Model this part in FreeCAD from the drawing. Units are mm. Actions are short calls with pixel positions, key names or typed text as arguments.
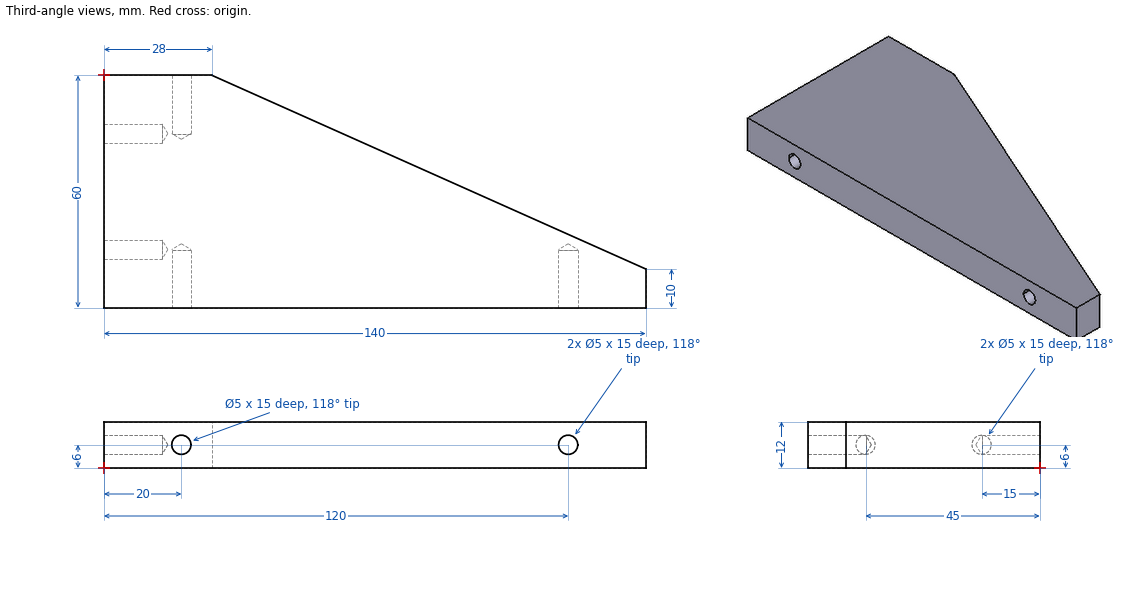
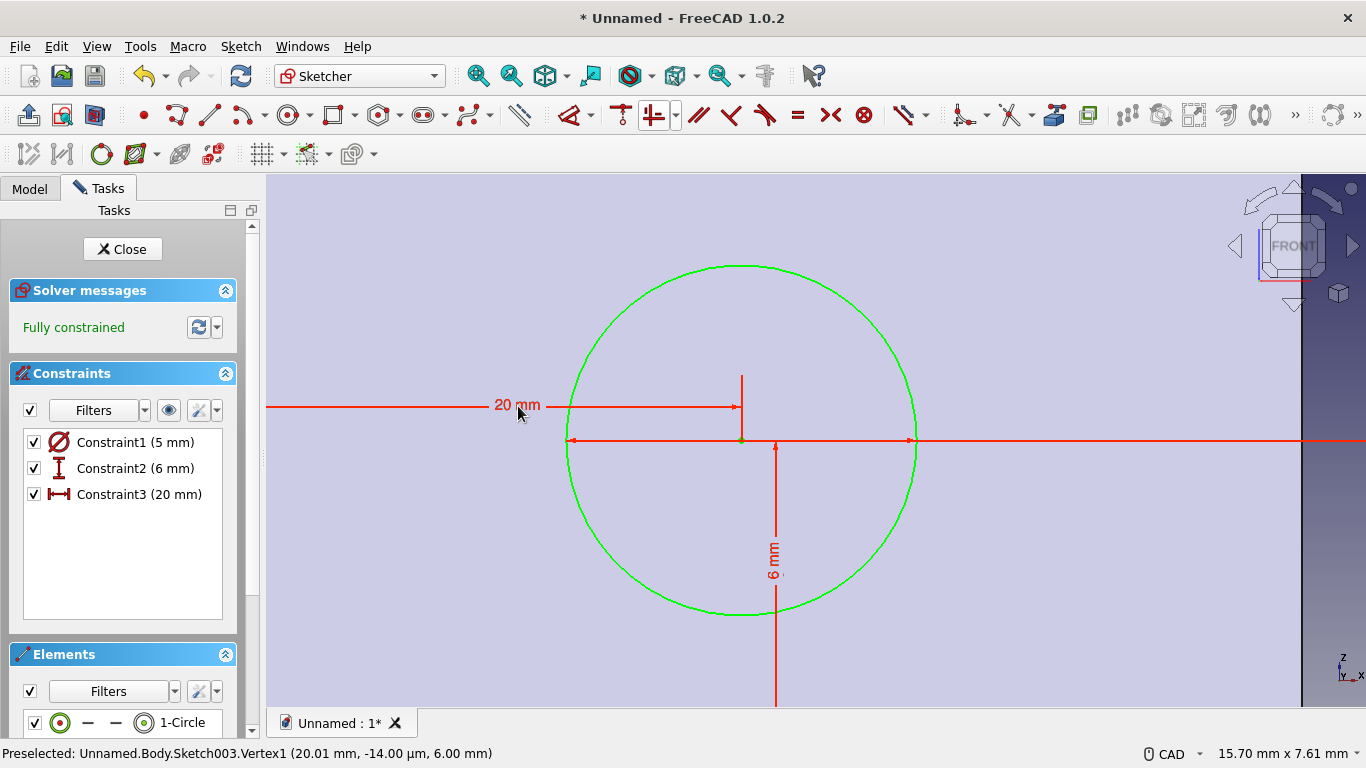
click(123, 249)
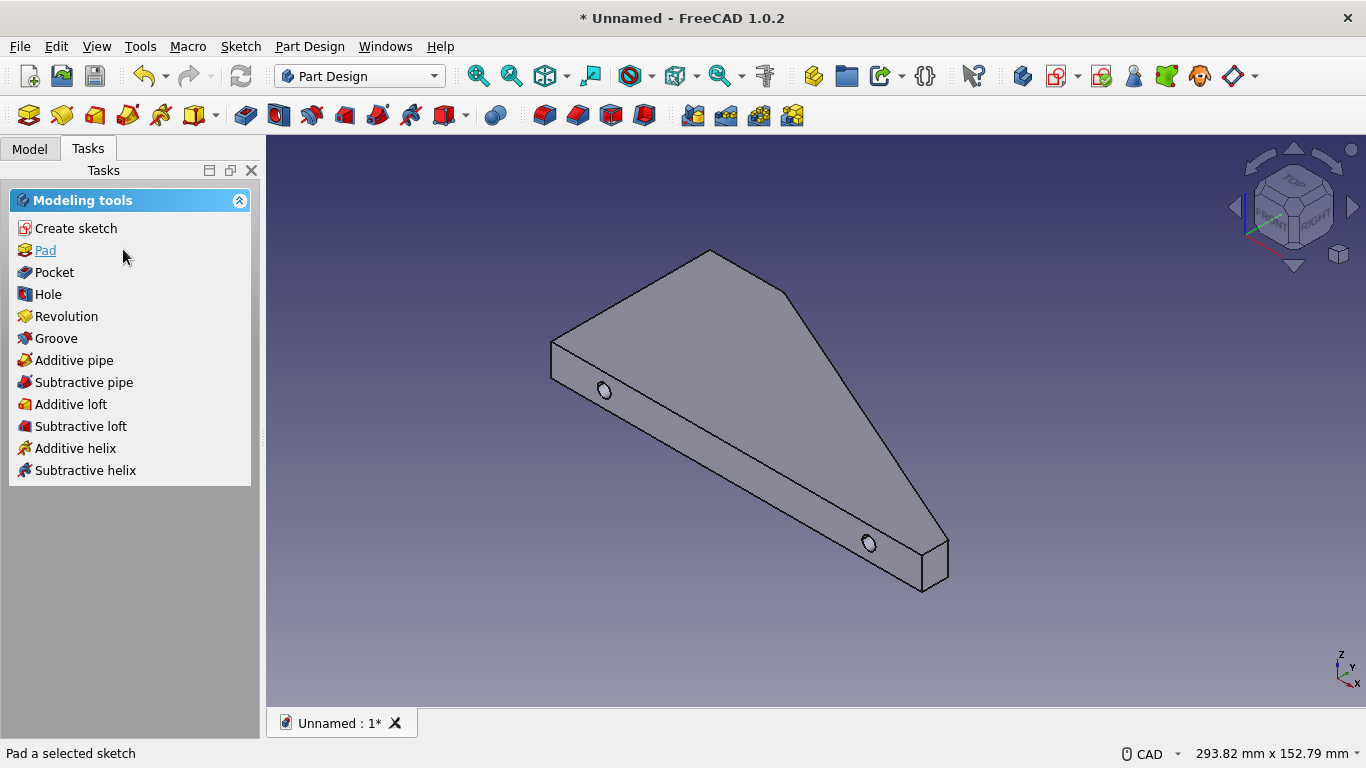
click(279, 116)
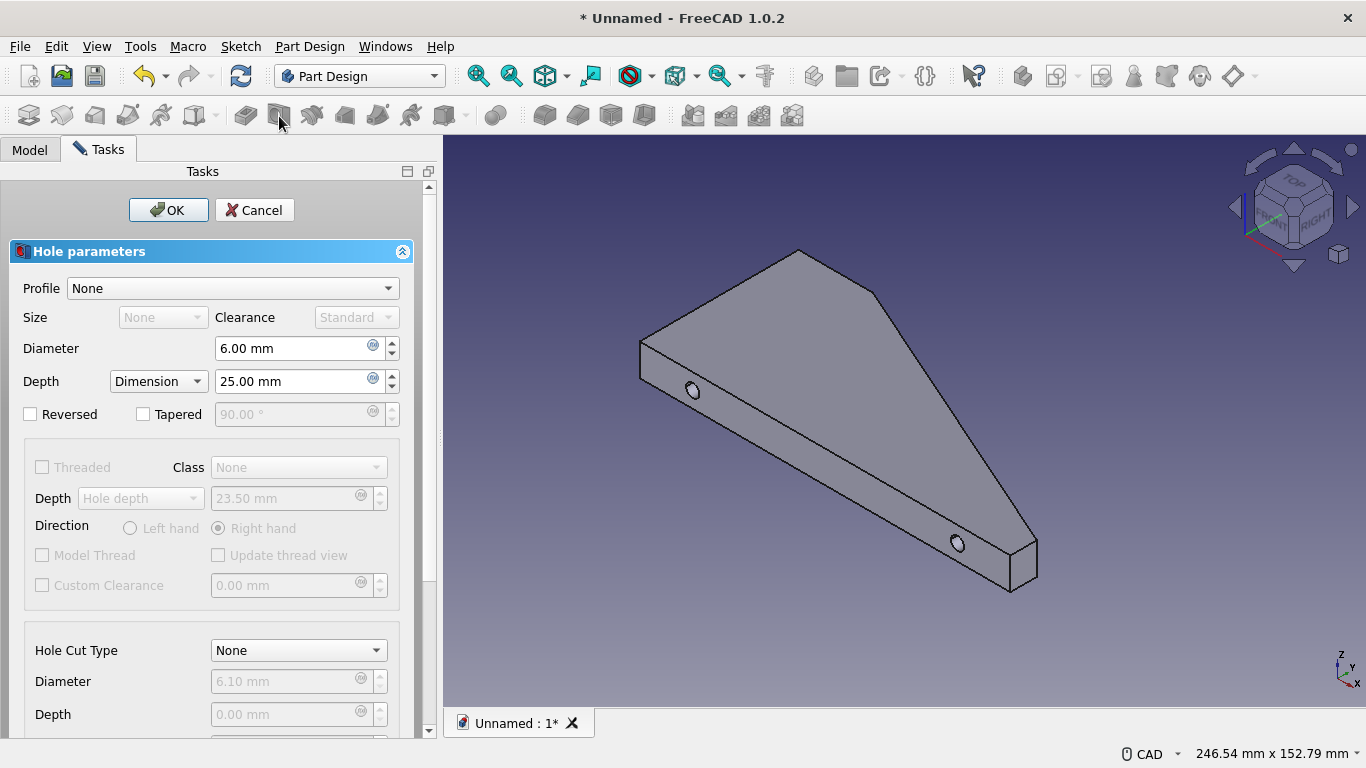
triple_click(300, 348)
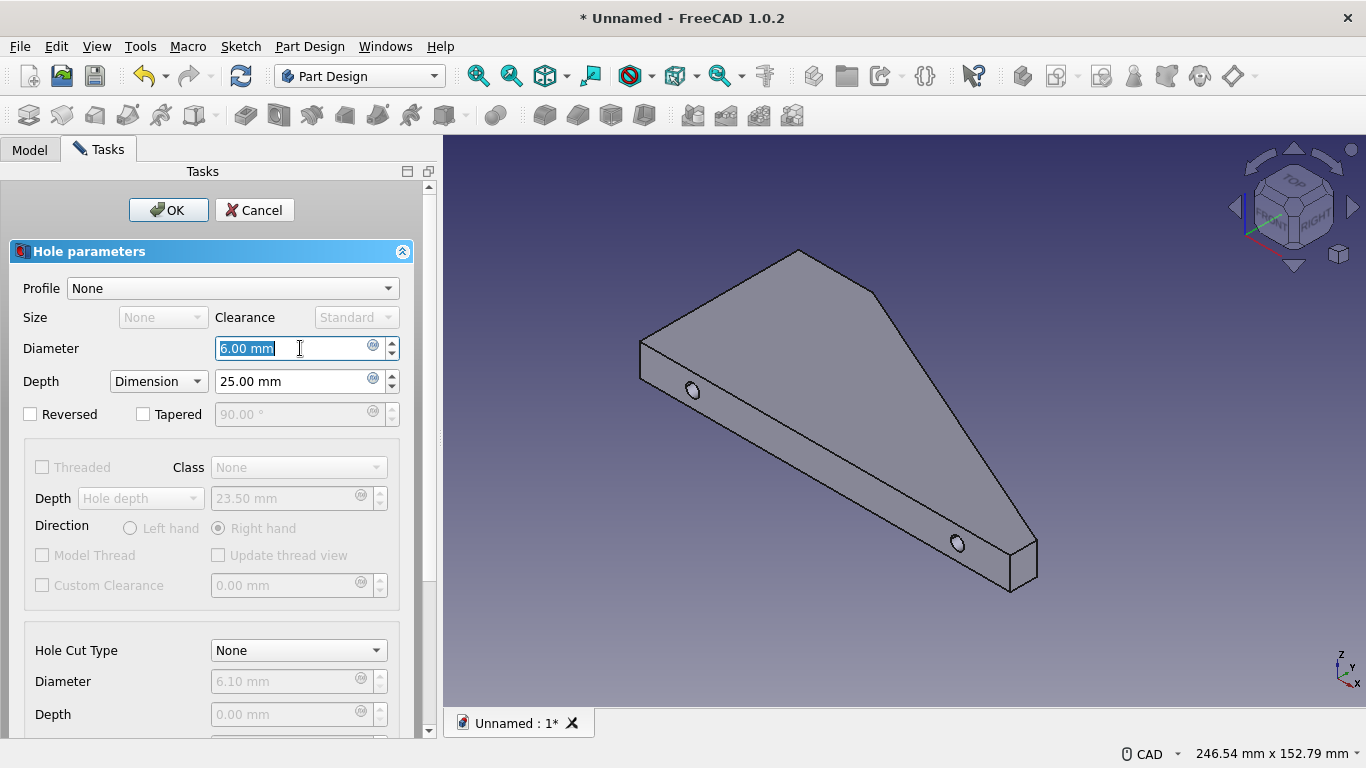
text(5)
key(Tab)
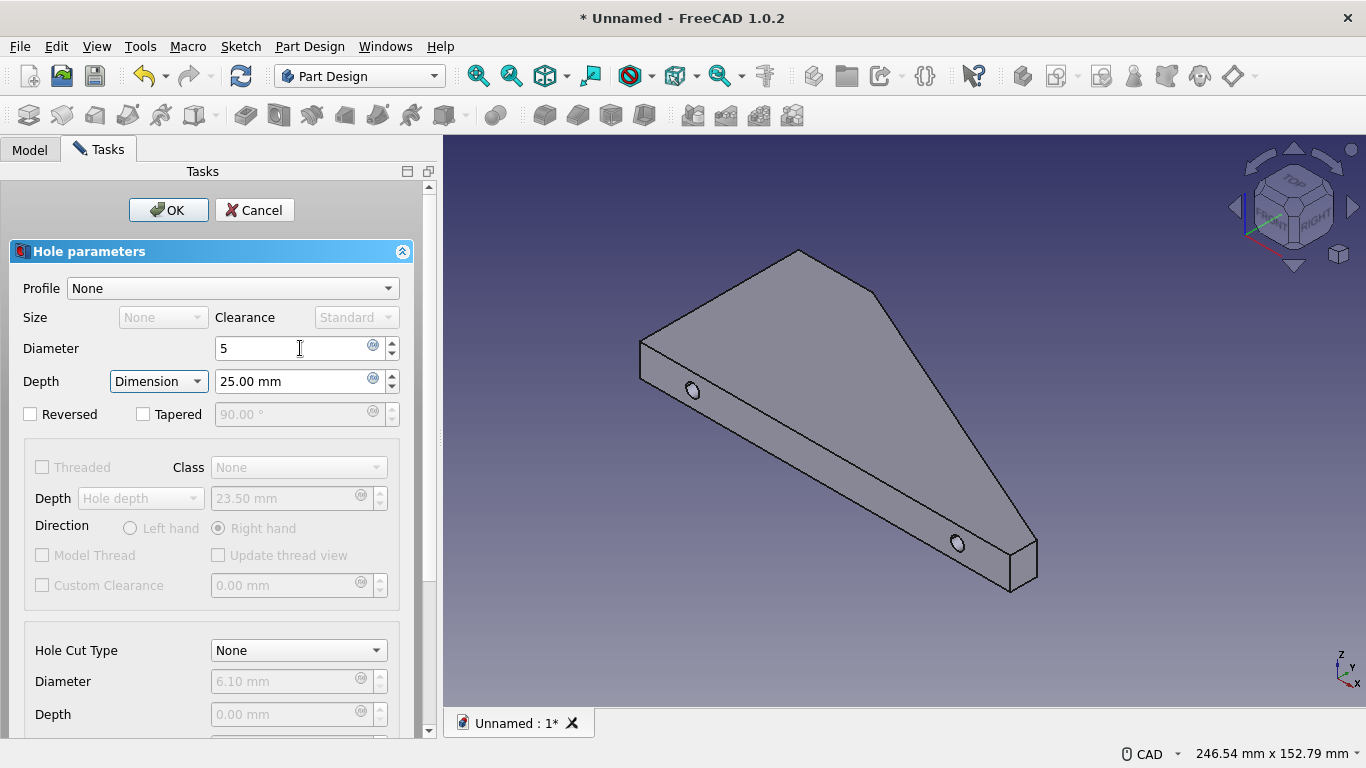
triple_click(300, 382)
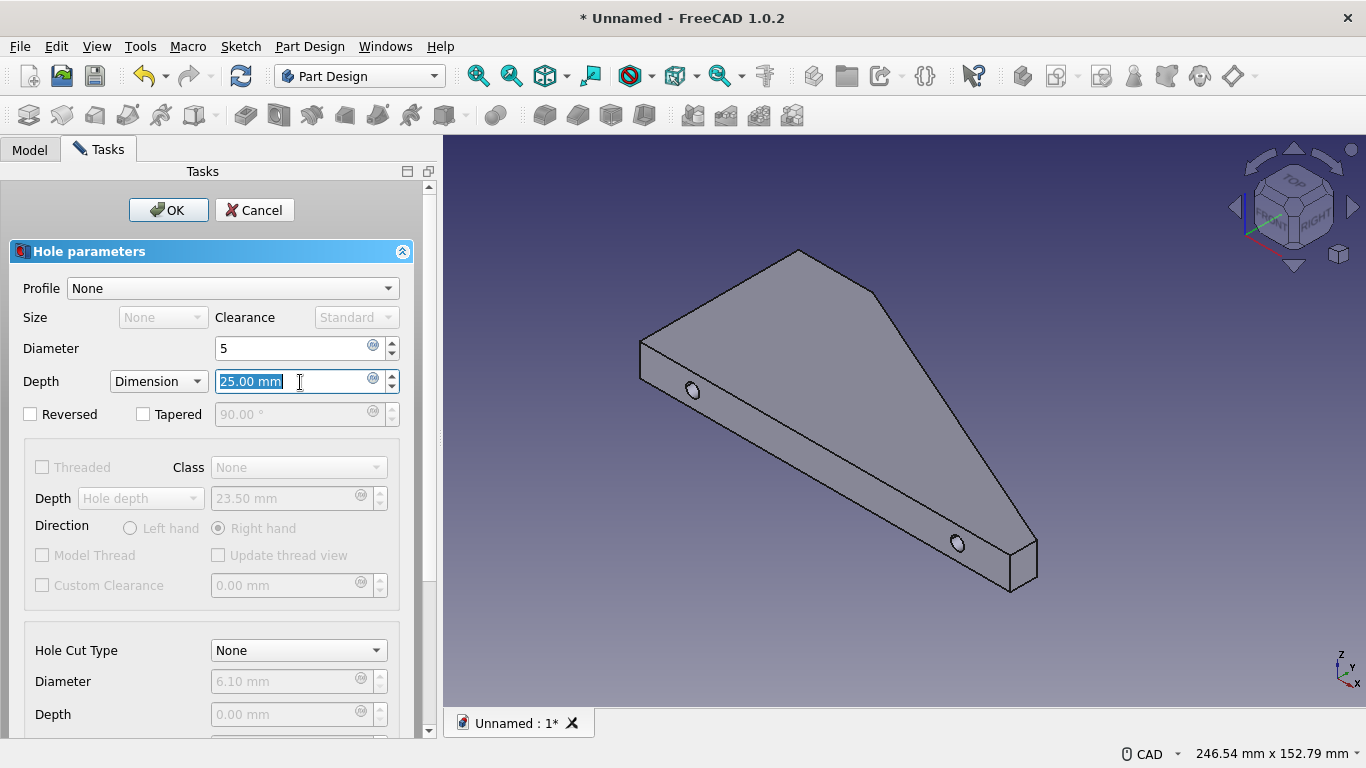
text(15)
key(Tab)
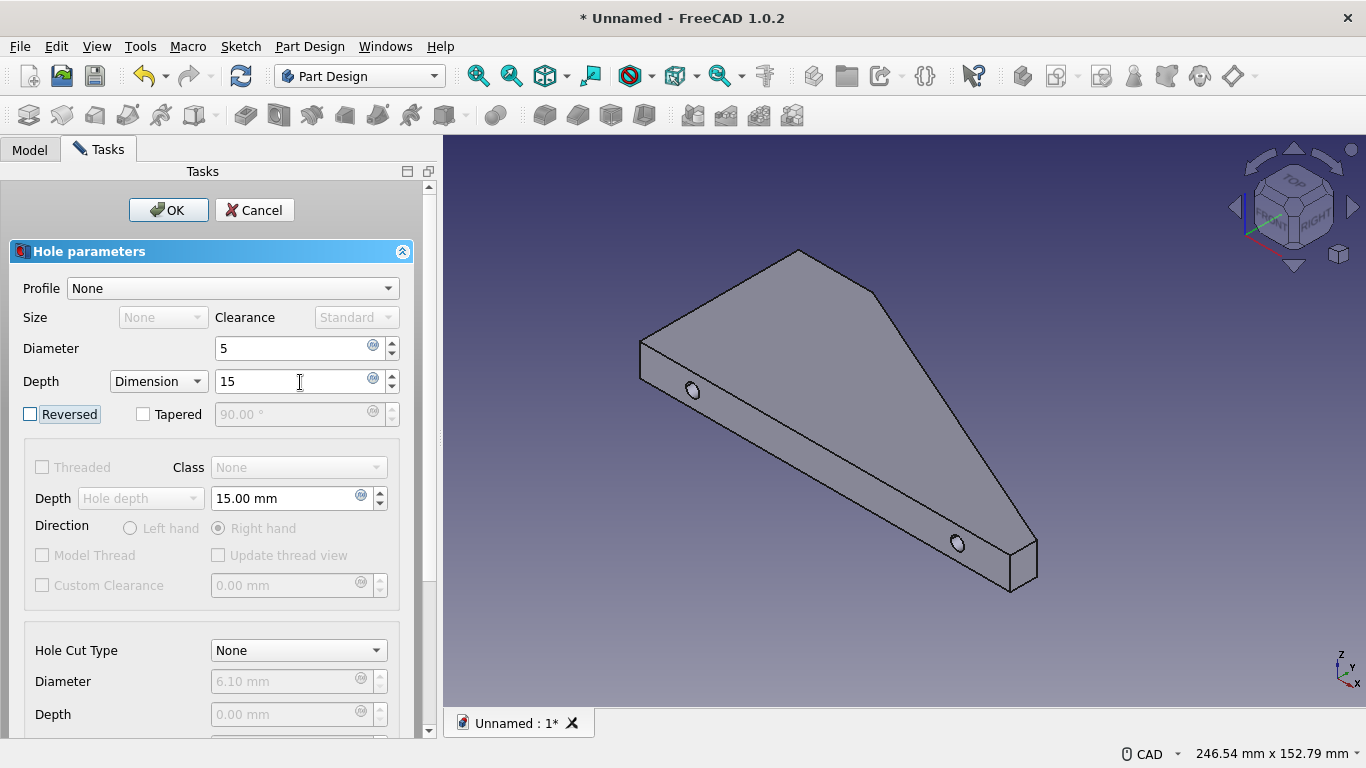
click(31, 414)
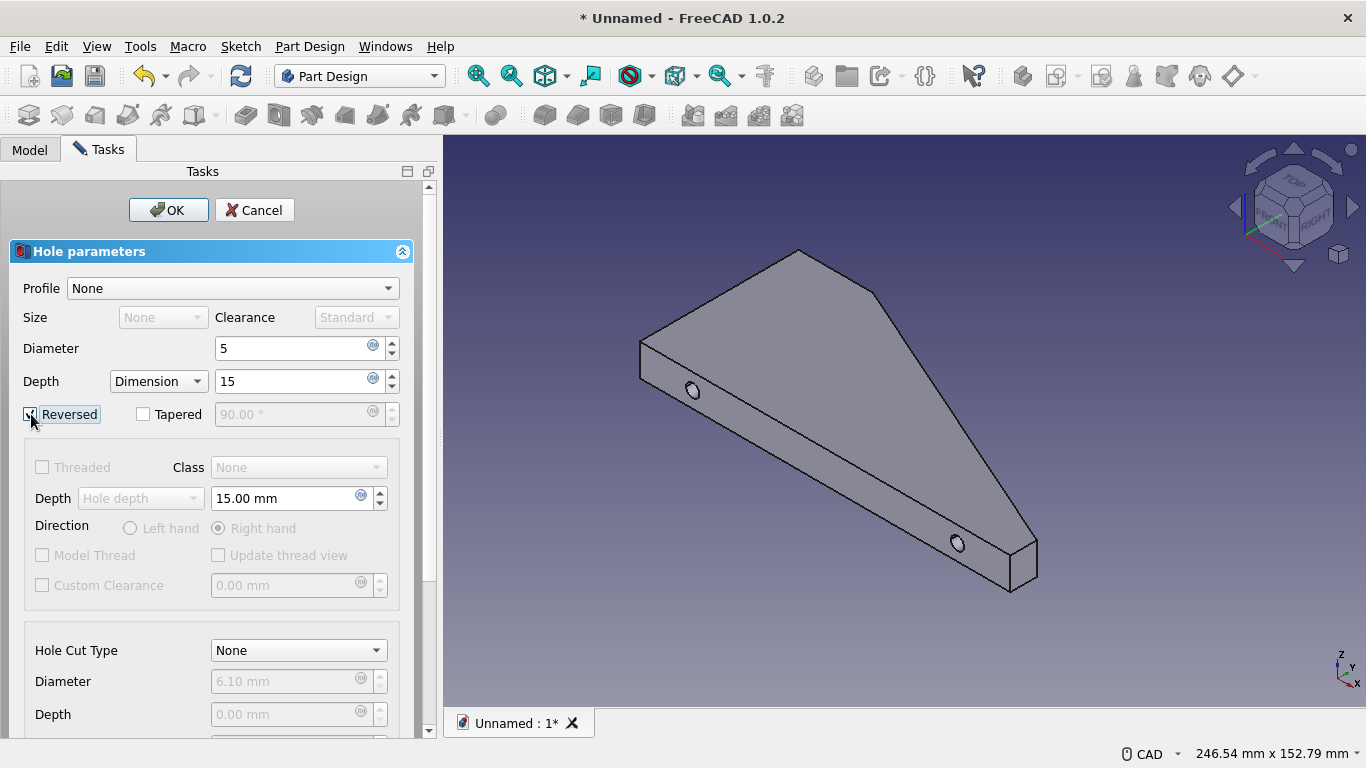
click(169, 210)